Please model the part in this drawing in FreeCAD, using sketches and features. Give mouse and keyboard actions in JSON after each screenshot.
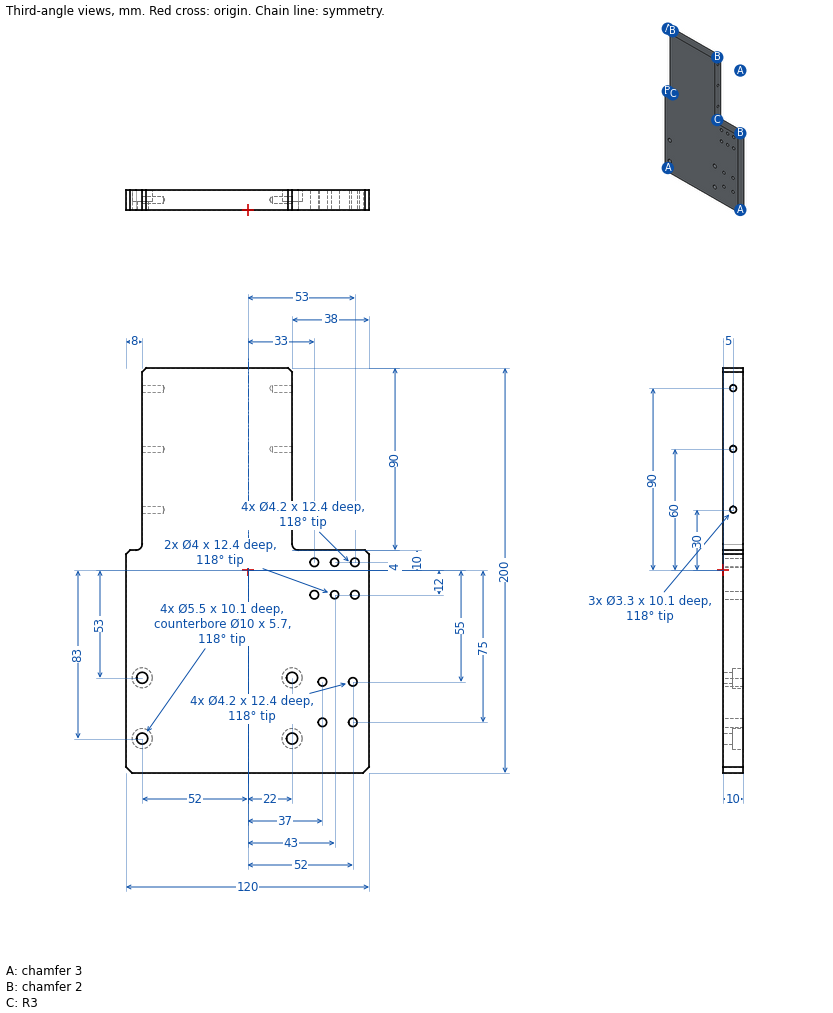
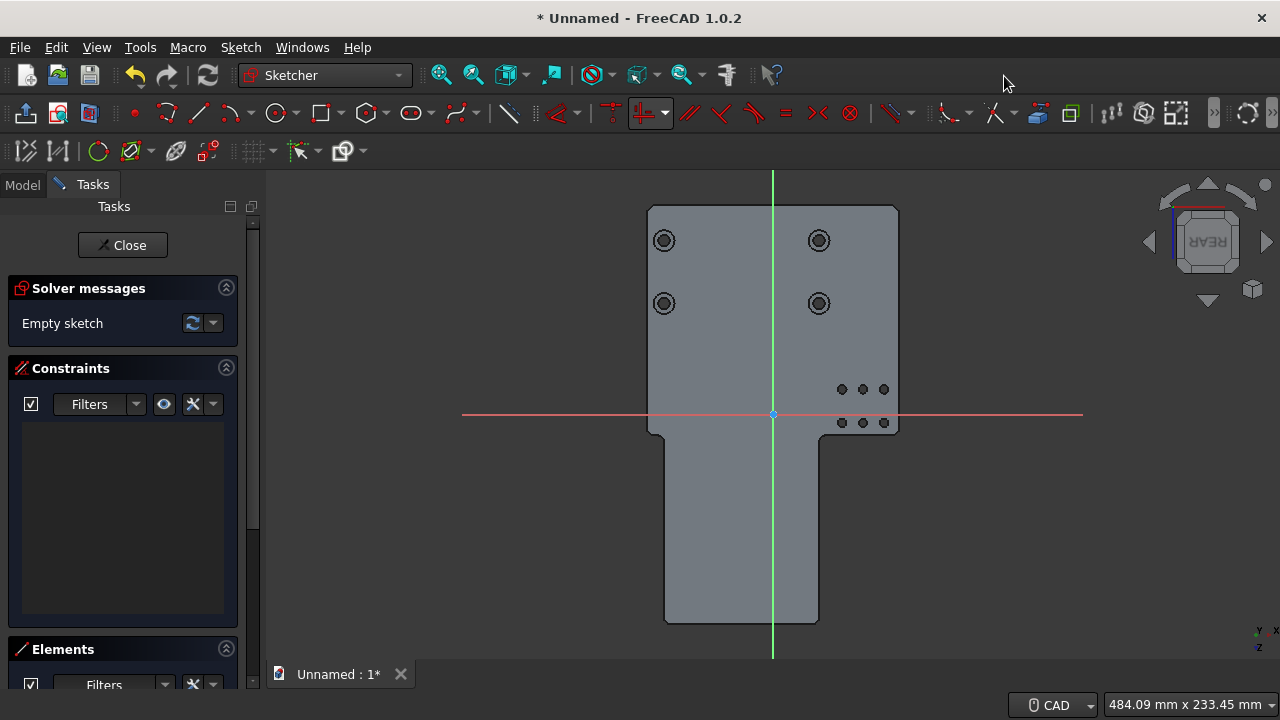
{"action": "scroll", "coordinate": [898, 251], "scroll_direction": "up", "scroll_amount": 9}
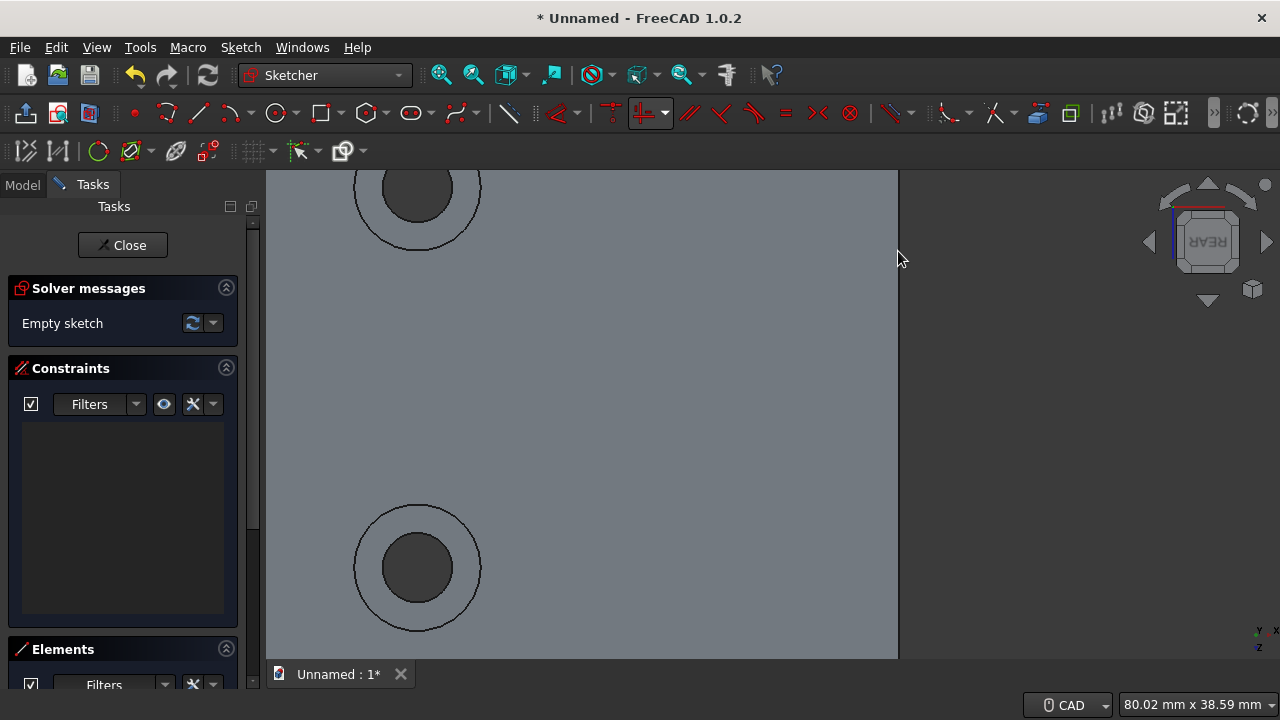
{"action": "left_click", "coordinate": [276, 114]}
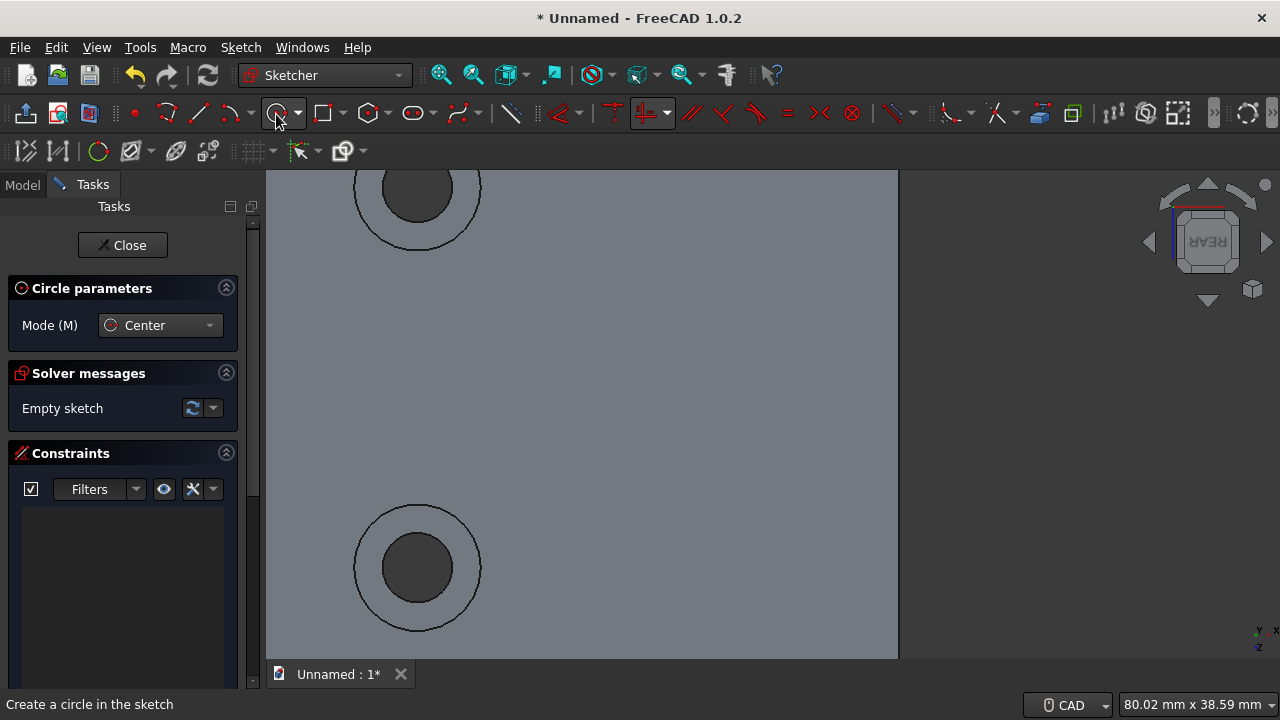
{"action": "left_click", "coordinate": [798, 542]}
{"action": "left_click", "coordinate": [816, 524]}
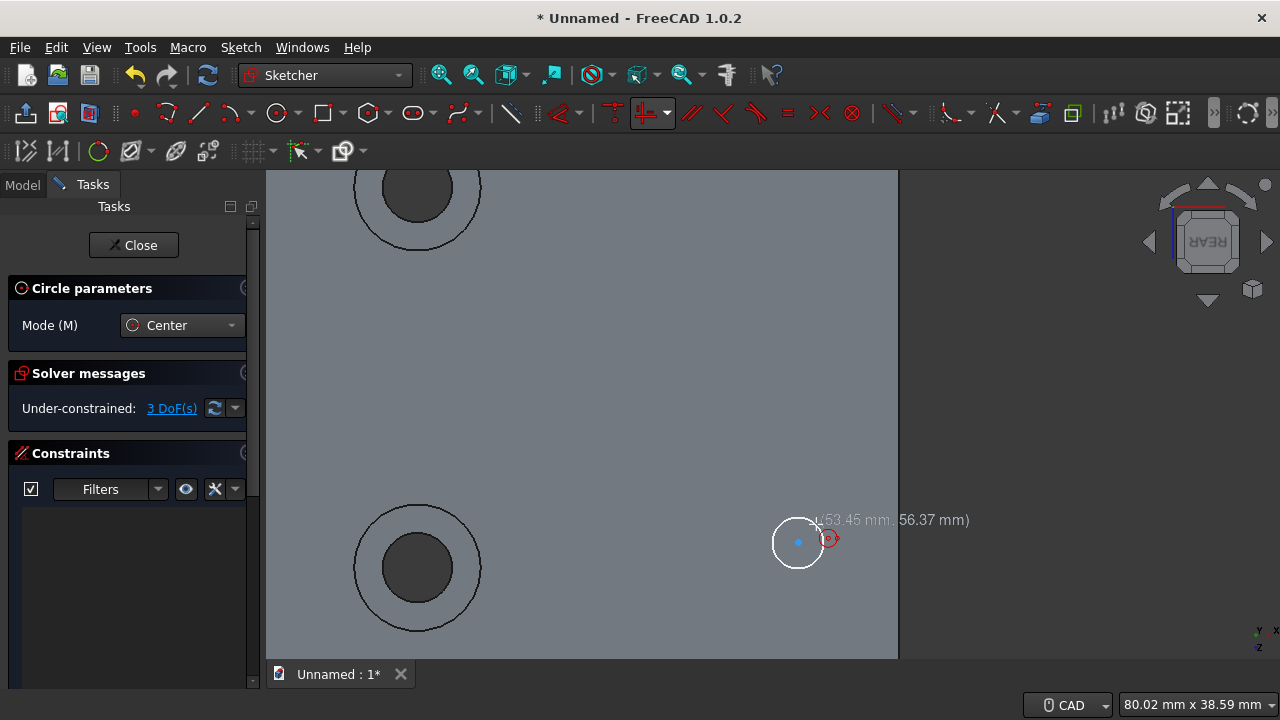
{"action": "left_click", "coordinate": [608, 542]}
{"action": "left_click", "coordinate": [626, 524]}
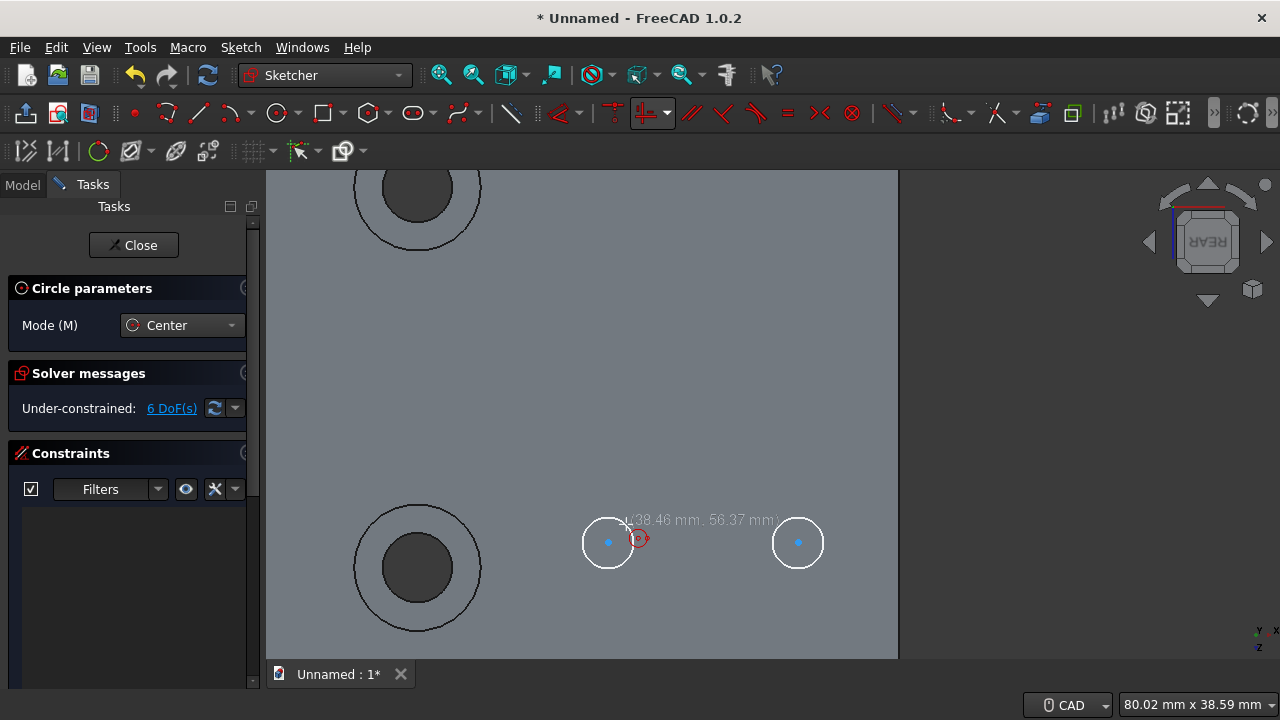
{"action": "left_click", "coordinate": [798, 289]}
{"action": "left_click", "coordinate": [816, 270]}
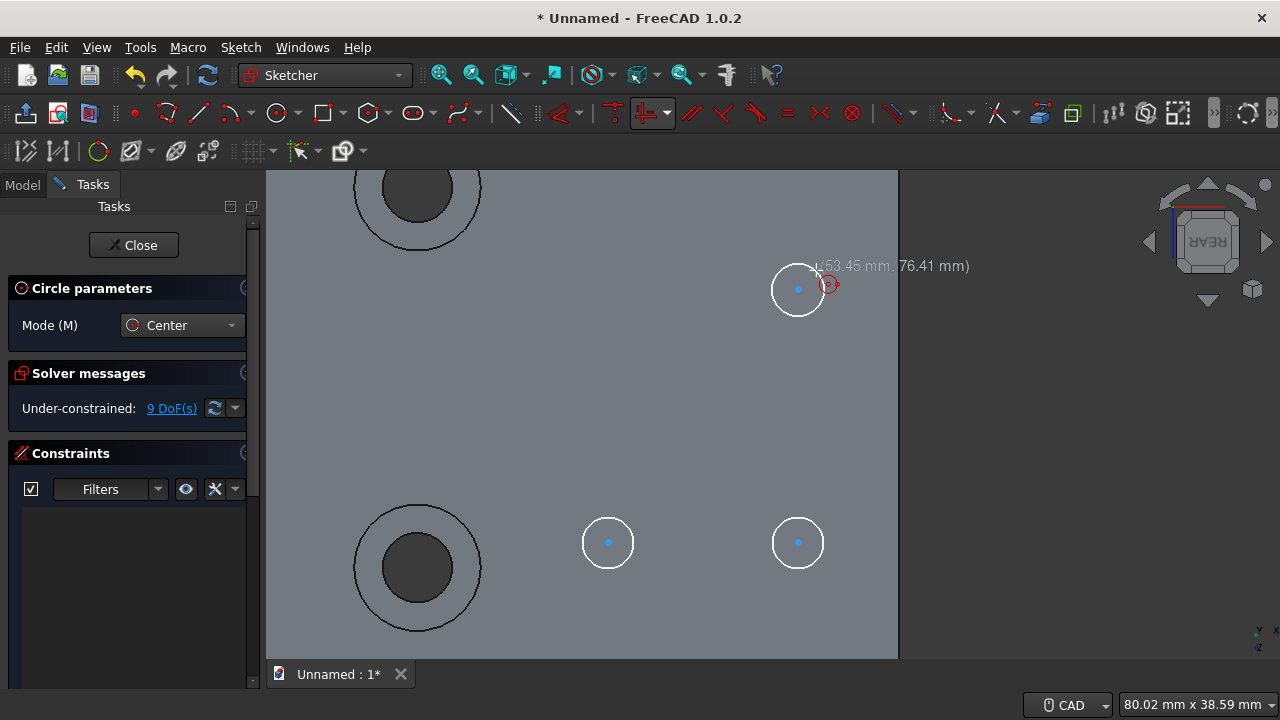
{"action": "left_click", "coordinate": [608, 289]}
{"action": "left_click", "coordinate": [626, 270]}
{"action": "key", "text": "Escape"}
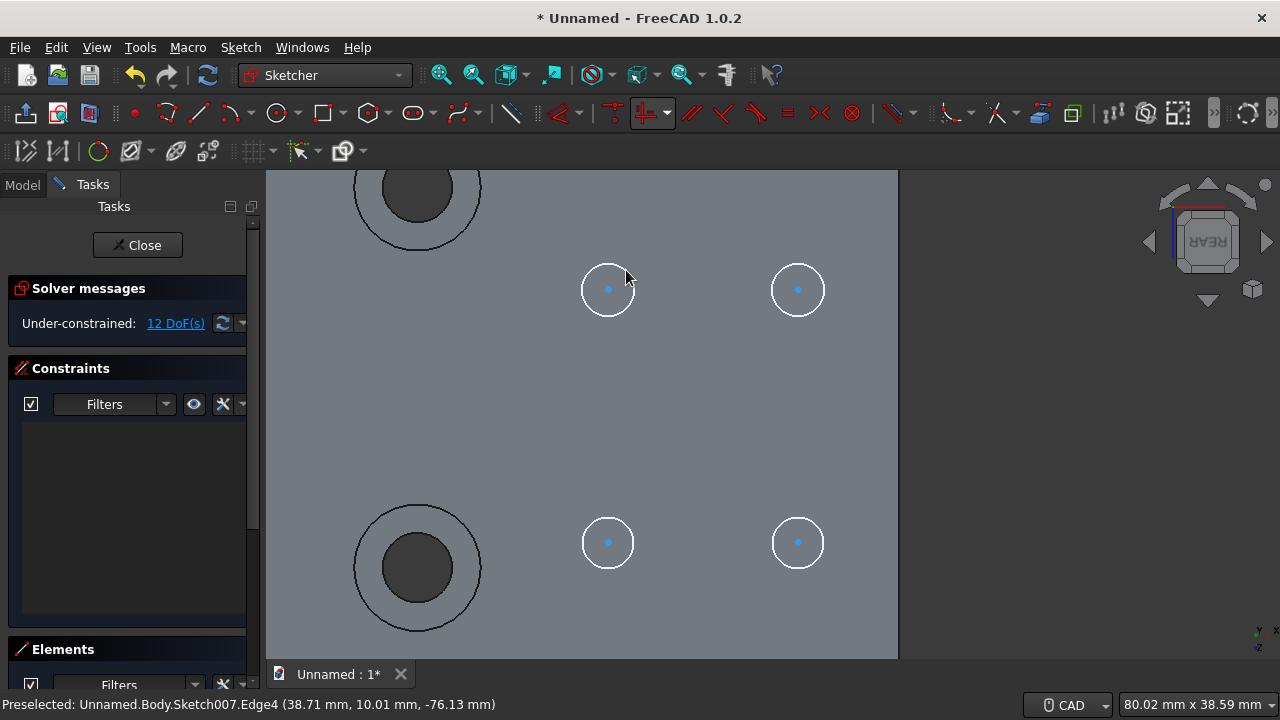
{"action": "left_click", "coordinate": [816, 525]}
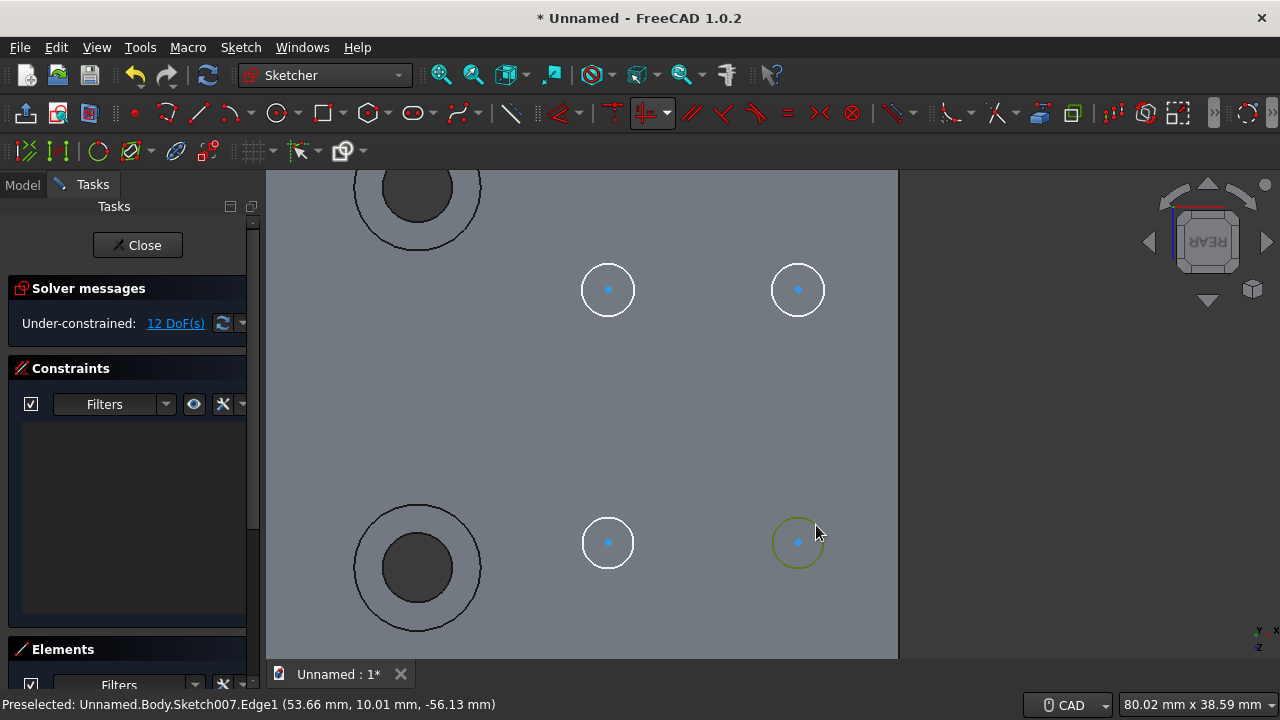
{"action": "left_click", "coordinate": [626, 525]}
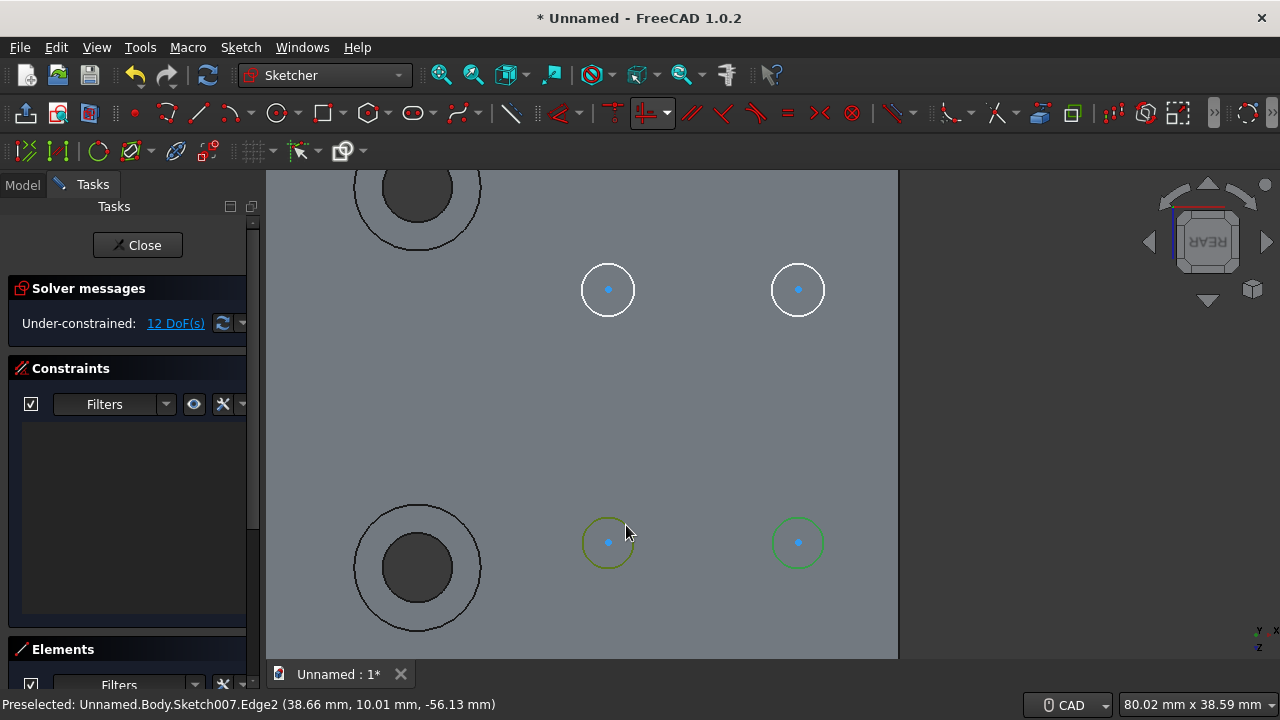
{"action": "left_click", "coordinate": [816, 271]}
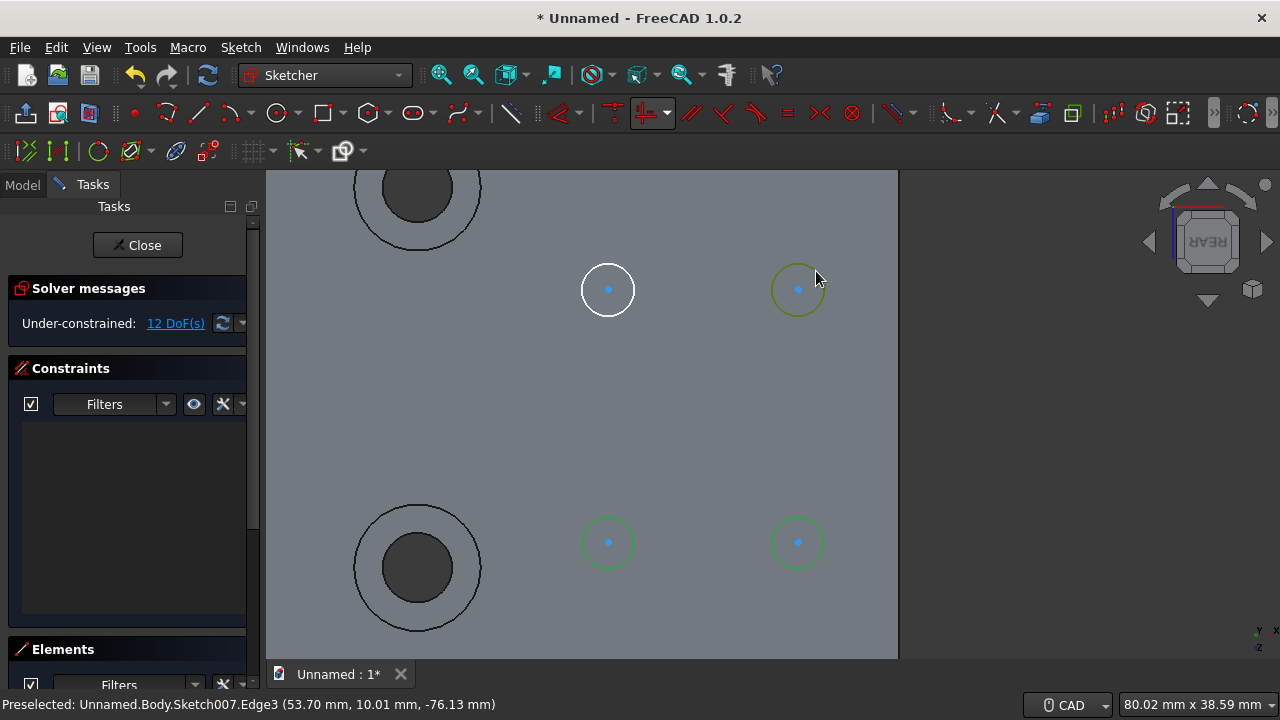
{"action": "left_click", "coordinate": [626, 271]}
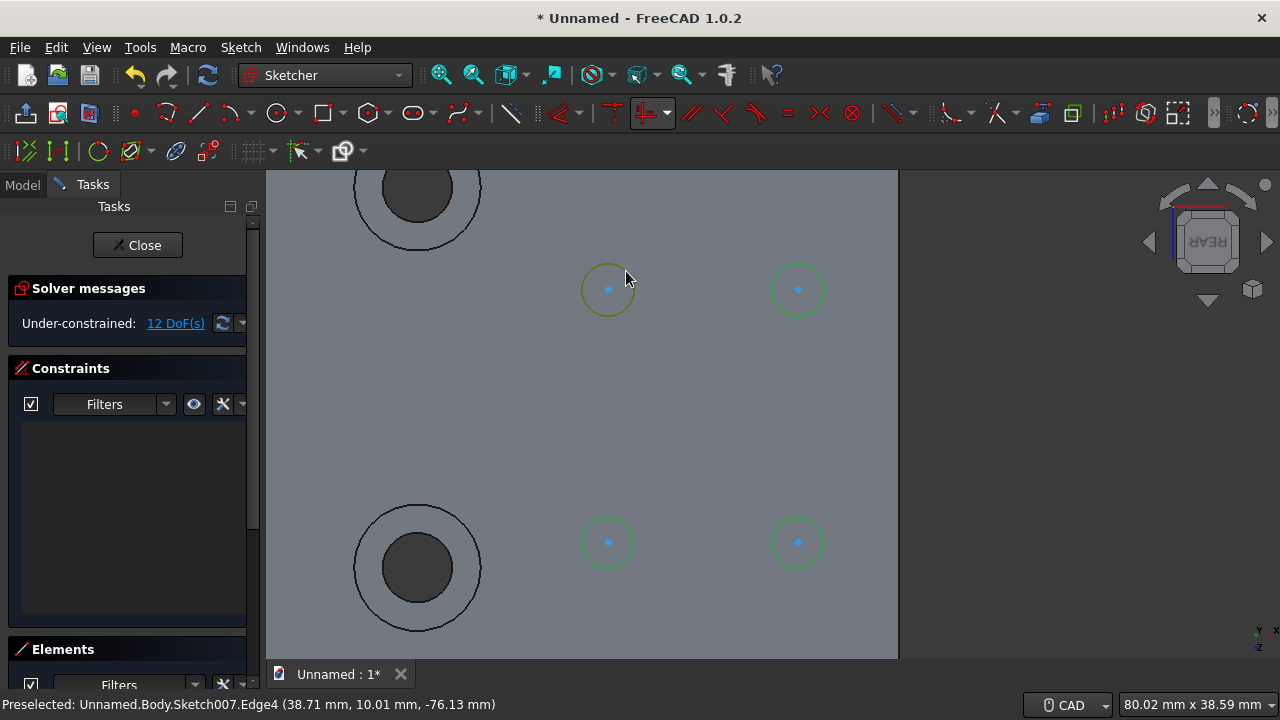
{"action": "left_click", "coordinate": [788, 114]}